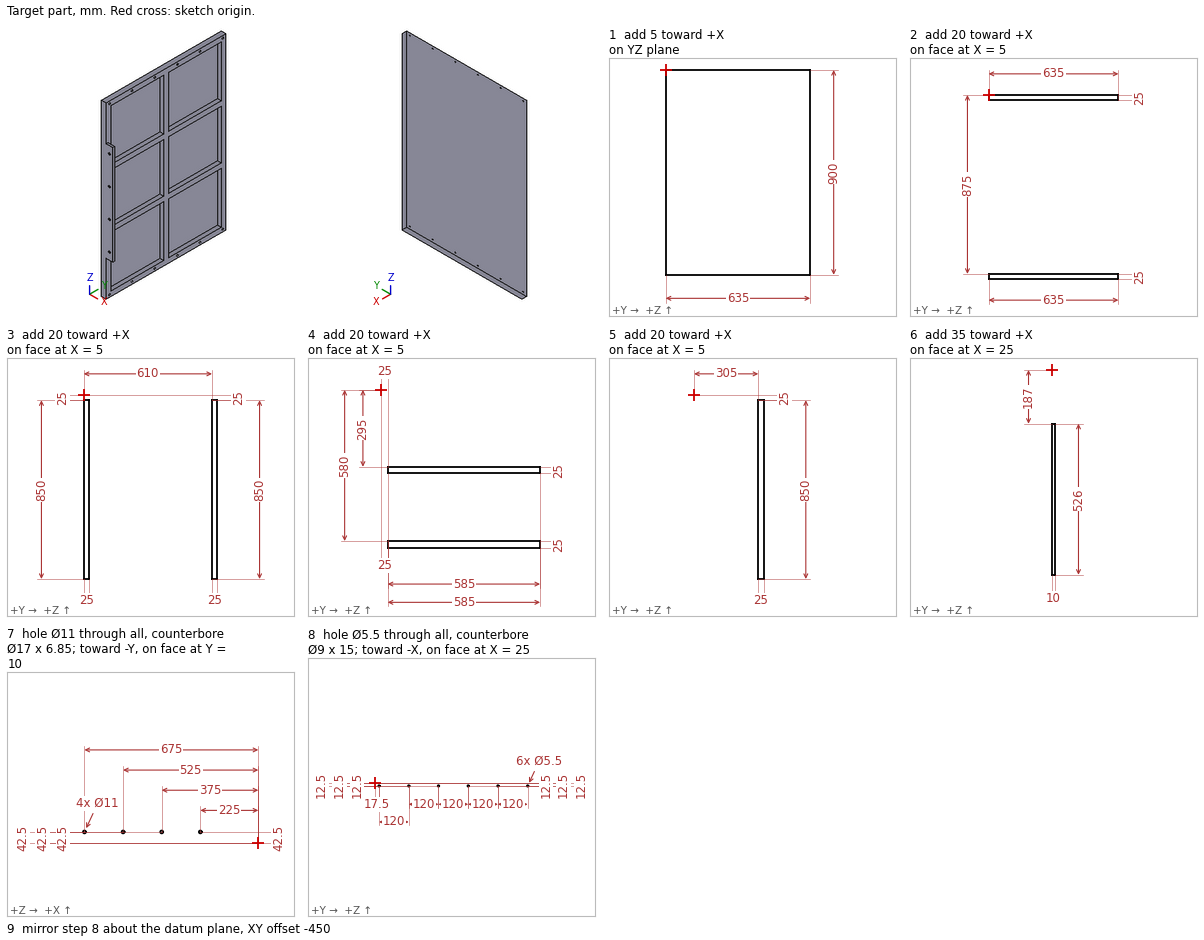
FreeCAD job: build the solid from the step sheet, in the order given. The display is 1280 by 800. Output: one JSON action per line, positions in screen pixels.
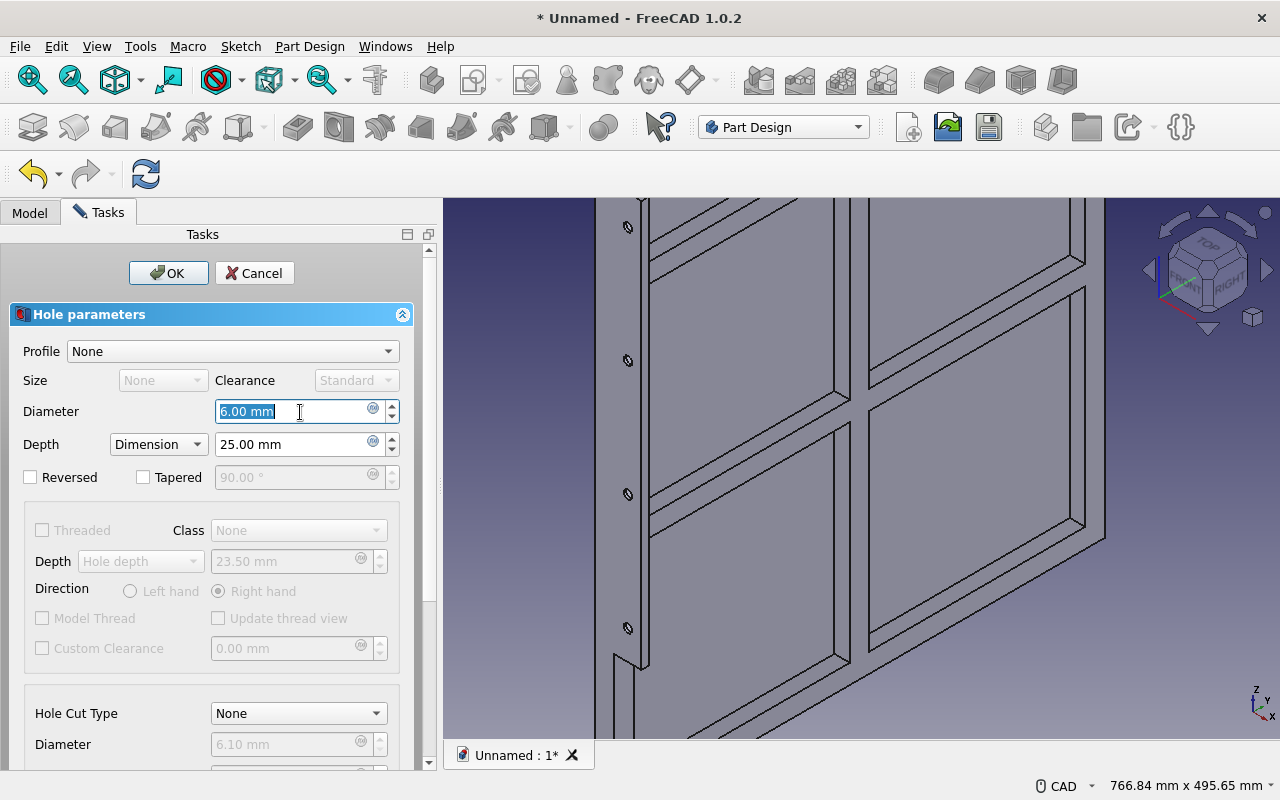
{"action": "type", "text": "5.5"}
{"action": "key", "text": "Tab"}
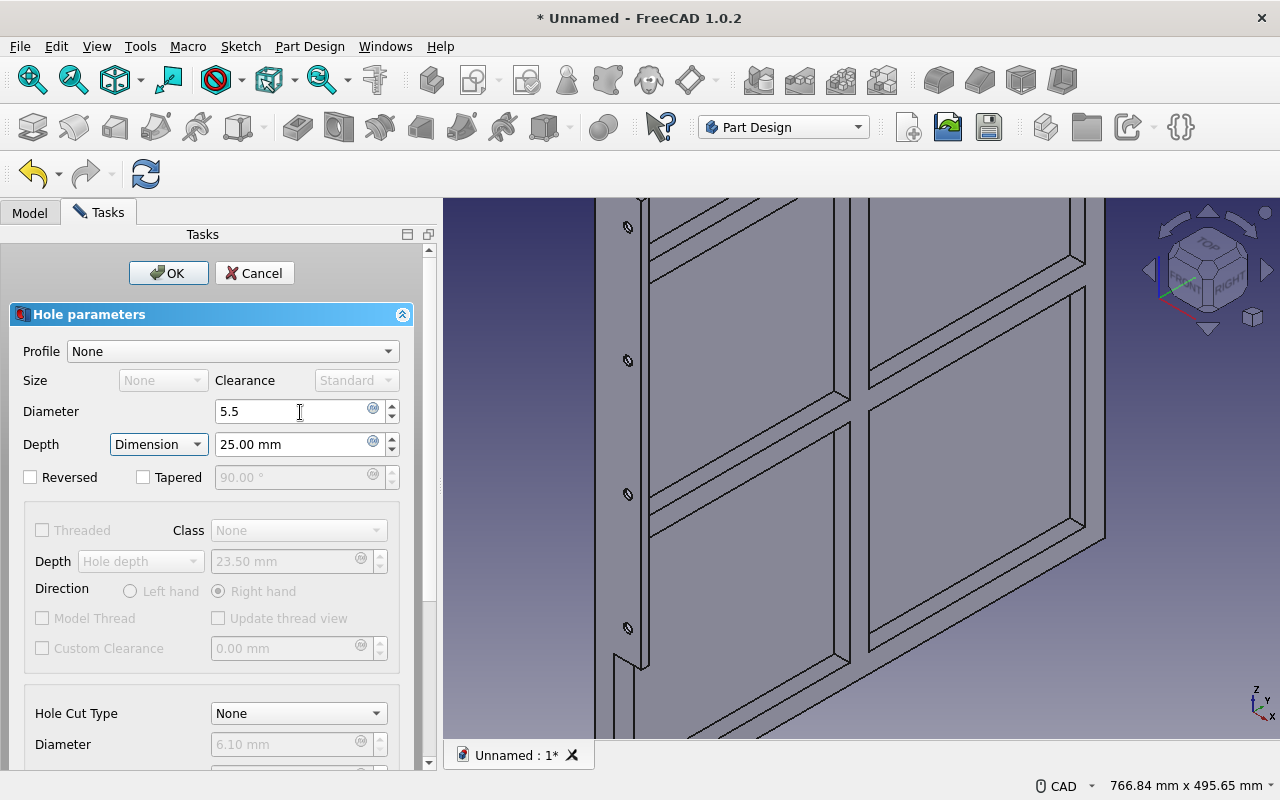
{"action": "left_click", "coordinate": [160, 444]}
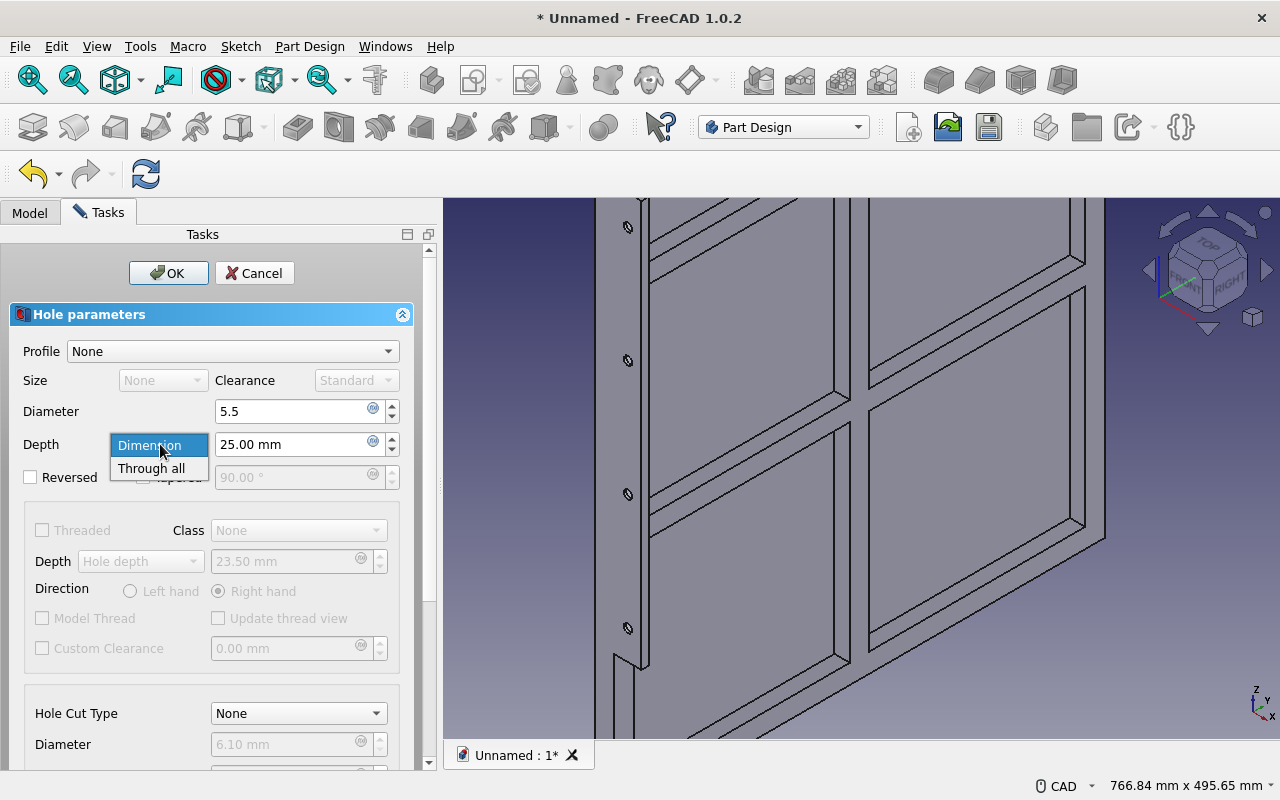
{"action": "left_click", "coordinate": [158, 468]}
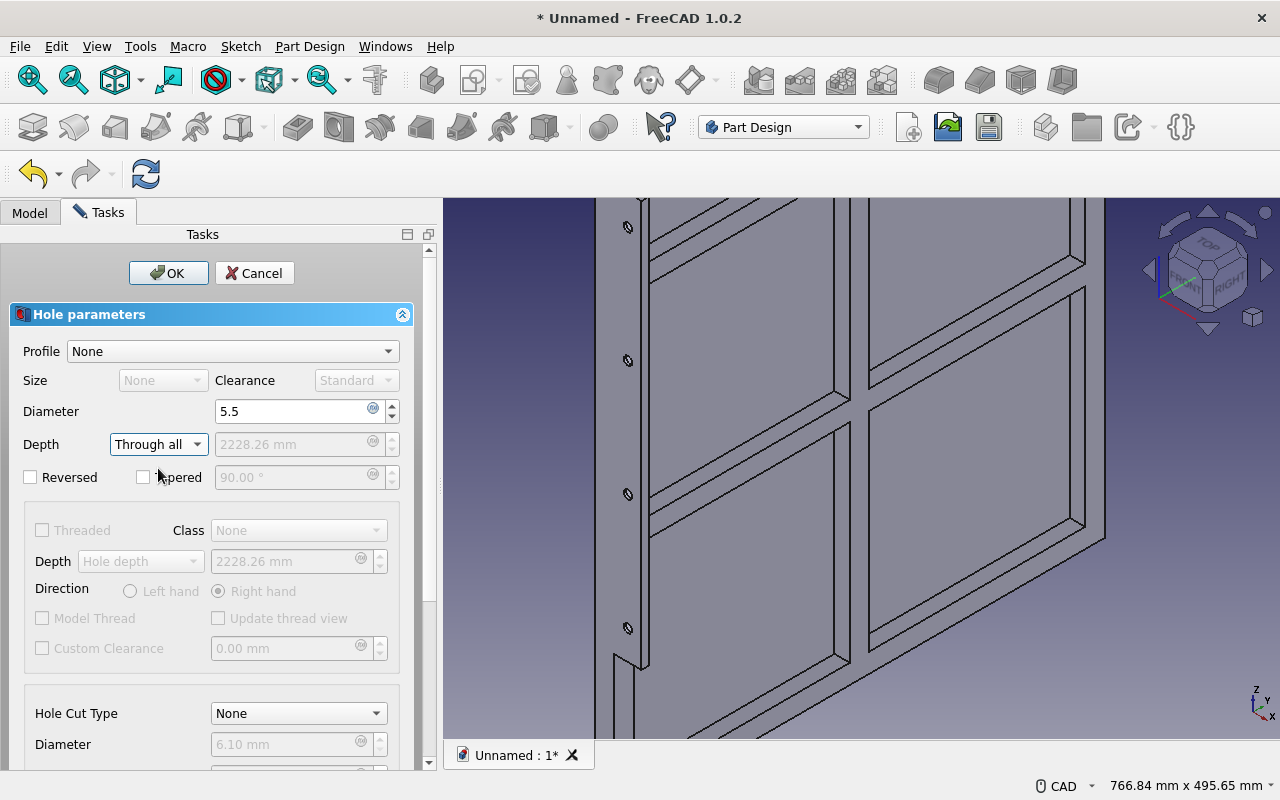
{"action": "left_click", "coordinate": [300, 714]}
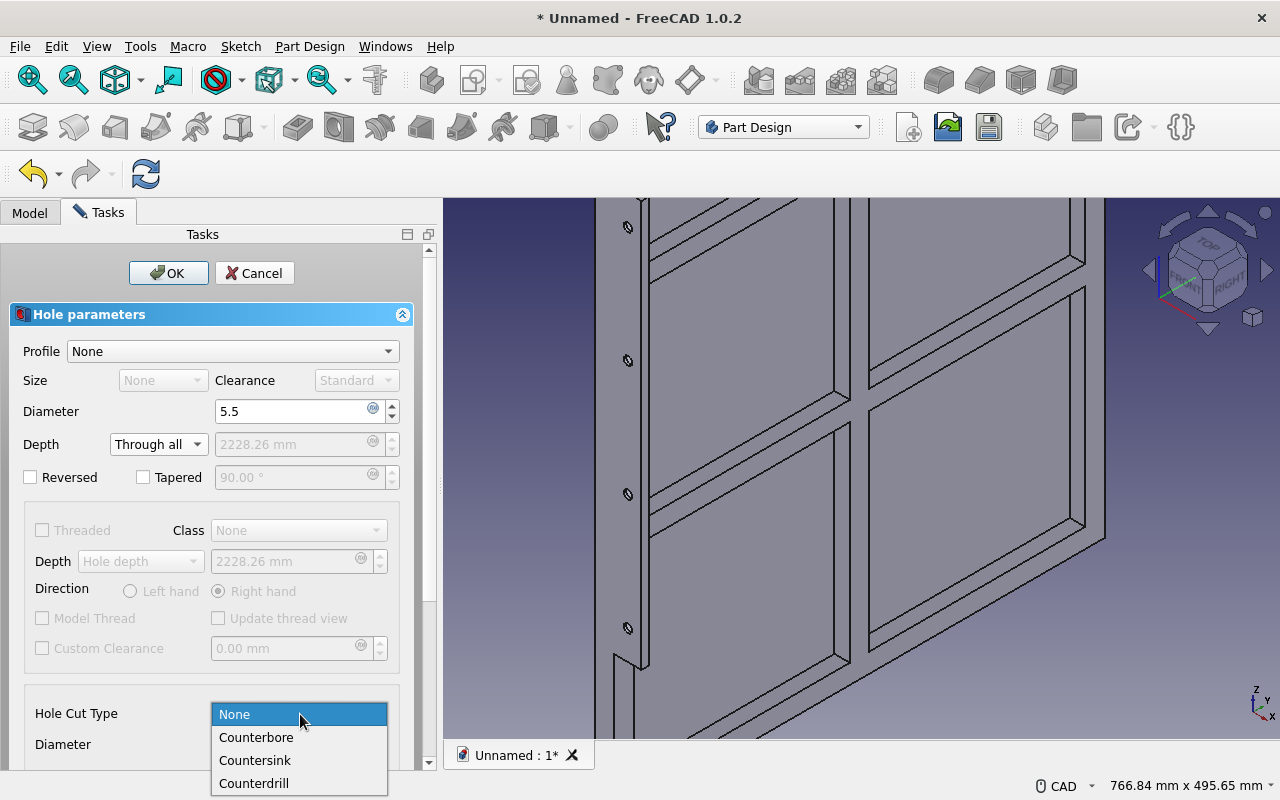
{"action": "left_click", "coordinate": [298, 738]}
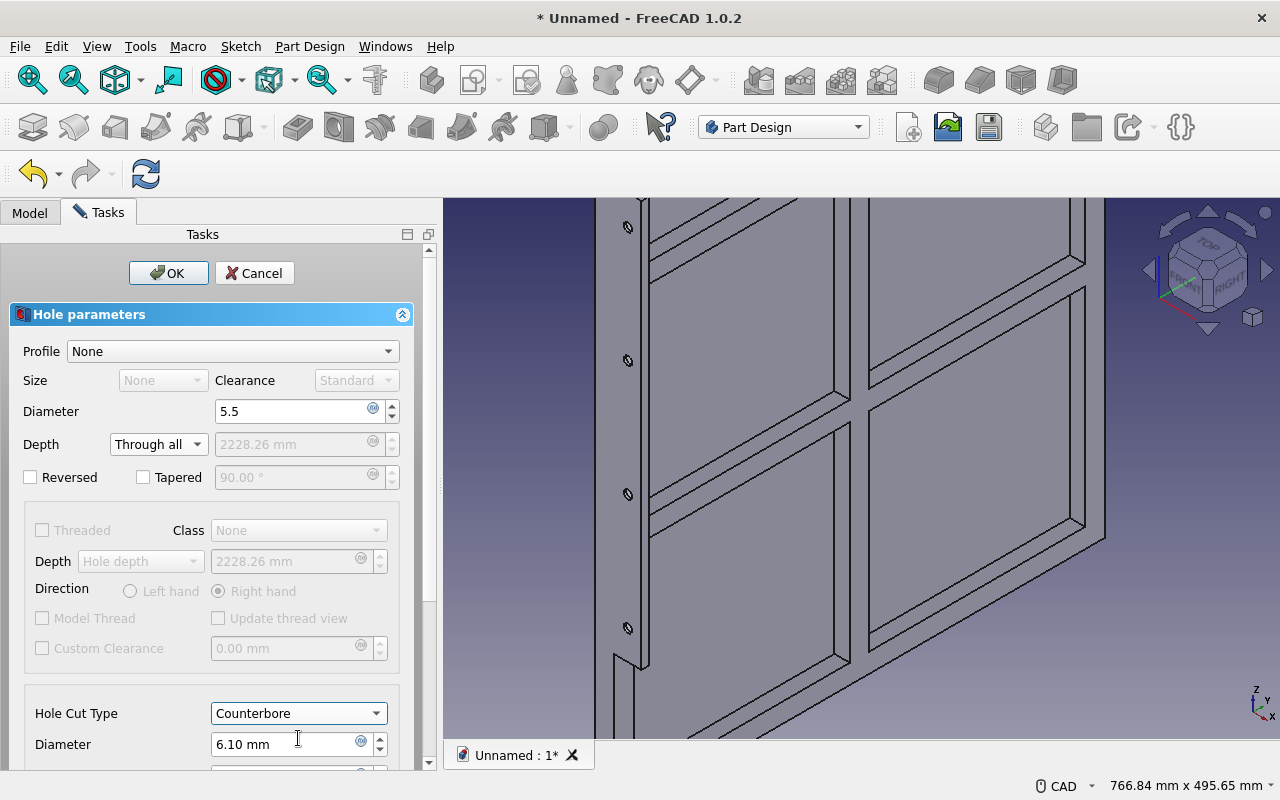
{"action": "triple_click", "coordinate": [292, 744]}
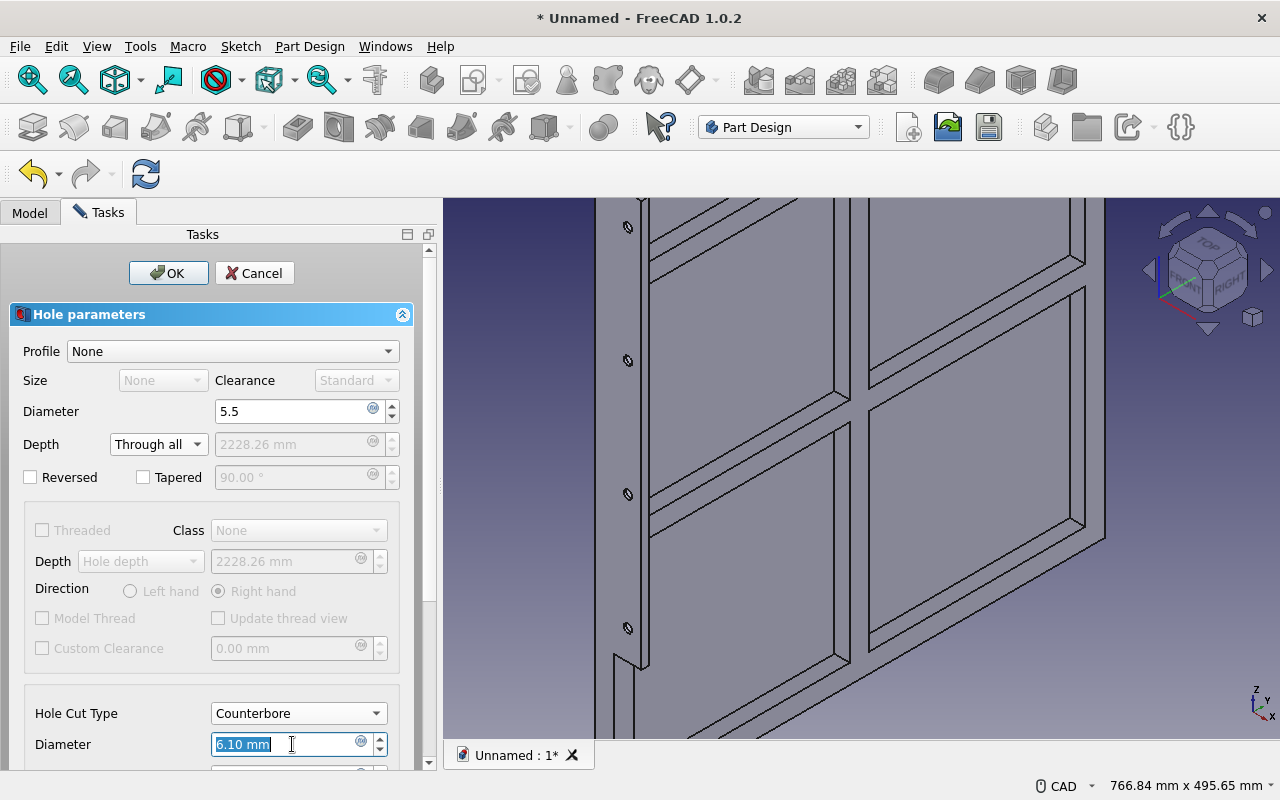
{"action": "type", "text": "9"}
{"action": "key", "text": "Tab"}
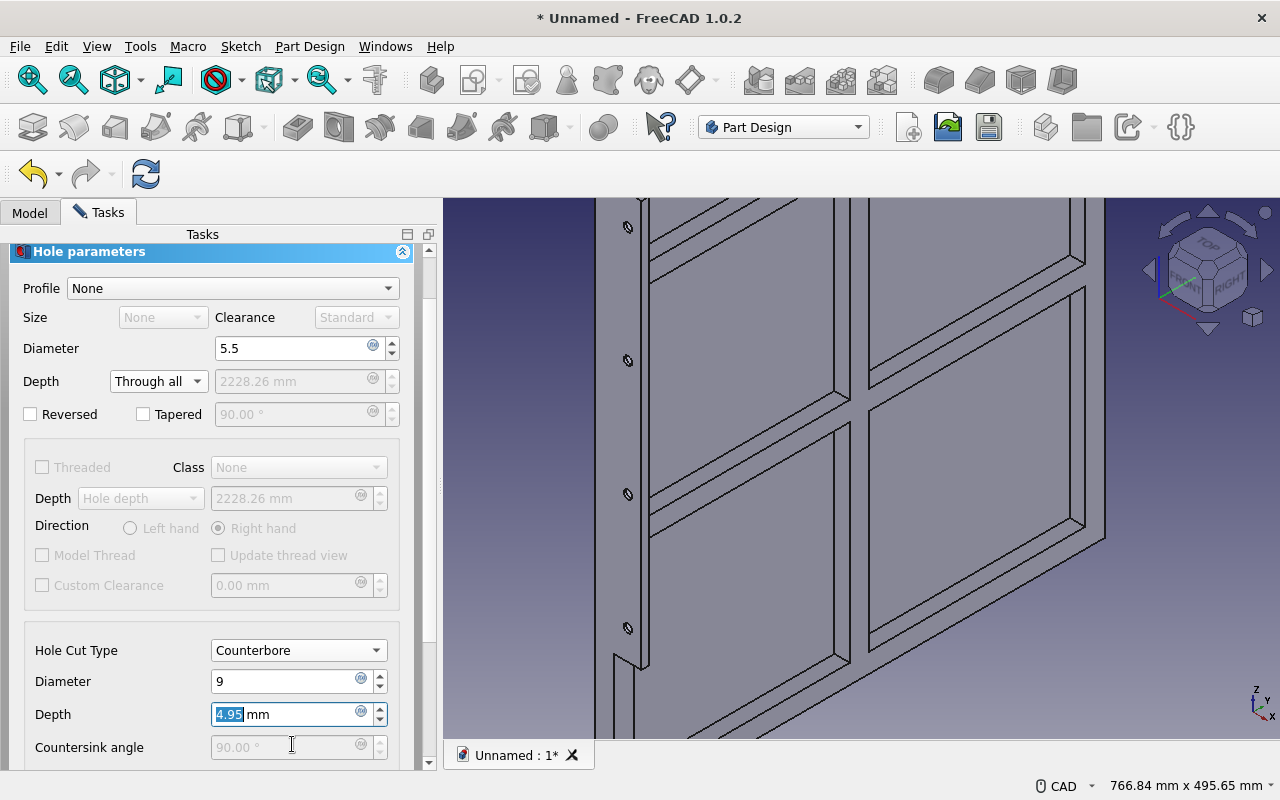
{"action": "type", "text": "15"}
{"action": "key", "text": "Tab"}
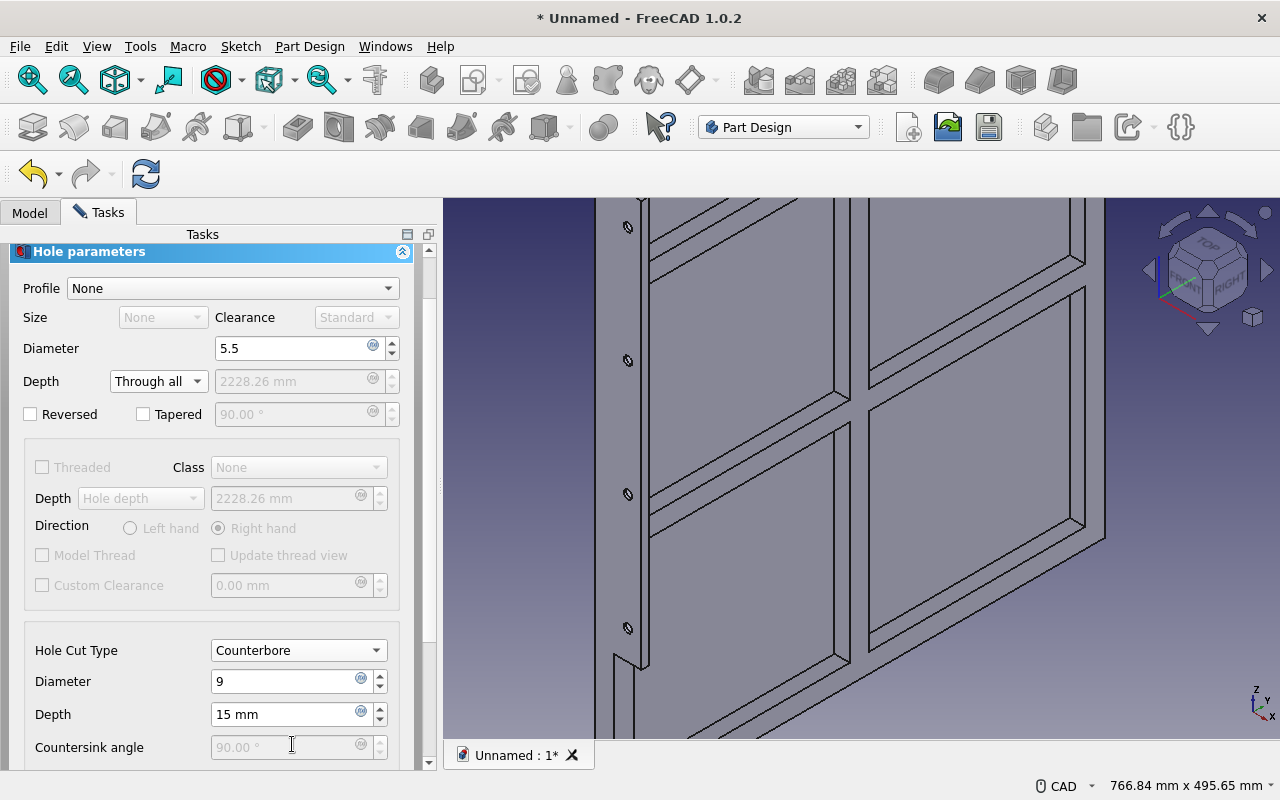
{"action": "scroll", "coordinate": [429, 507], "scroll_direction": "up", "scroll_amount": 2}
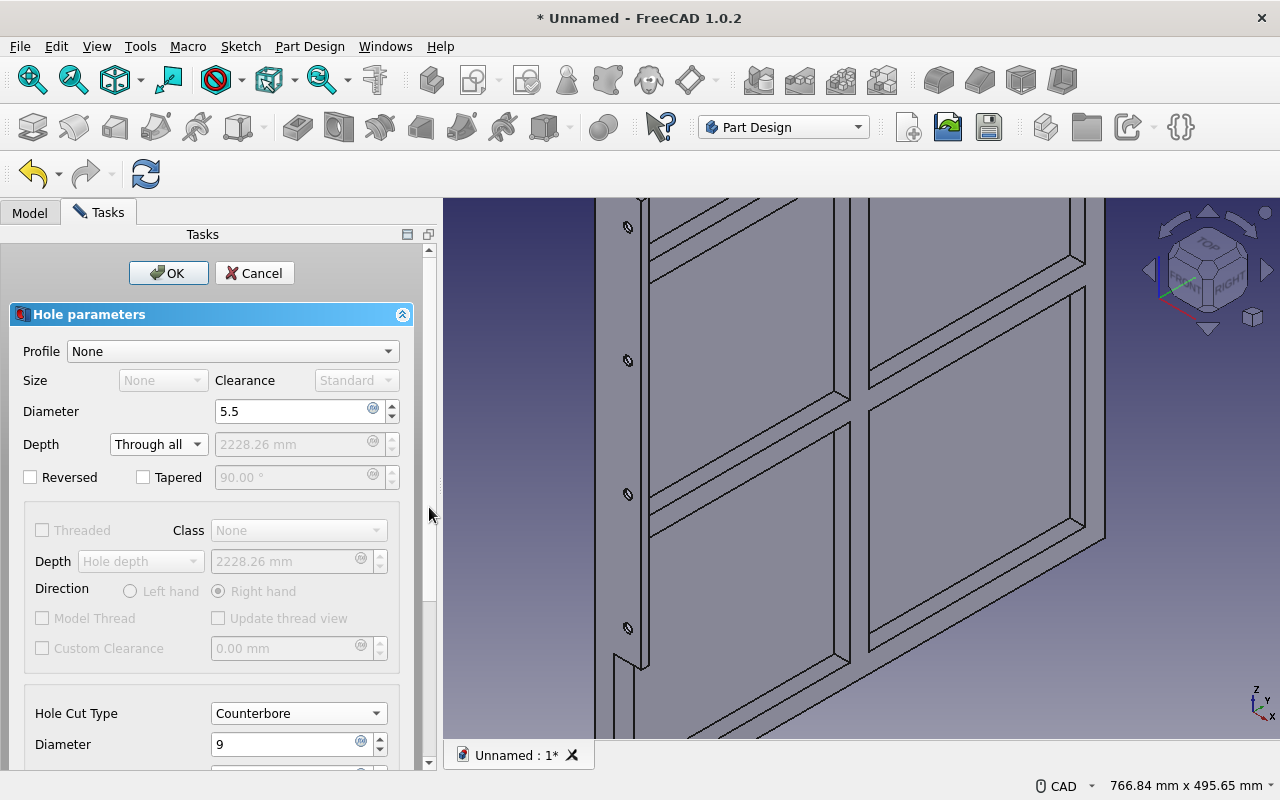
{"action": "left_click", "coordinate": [169, 273]}